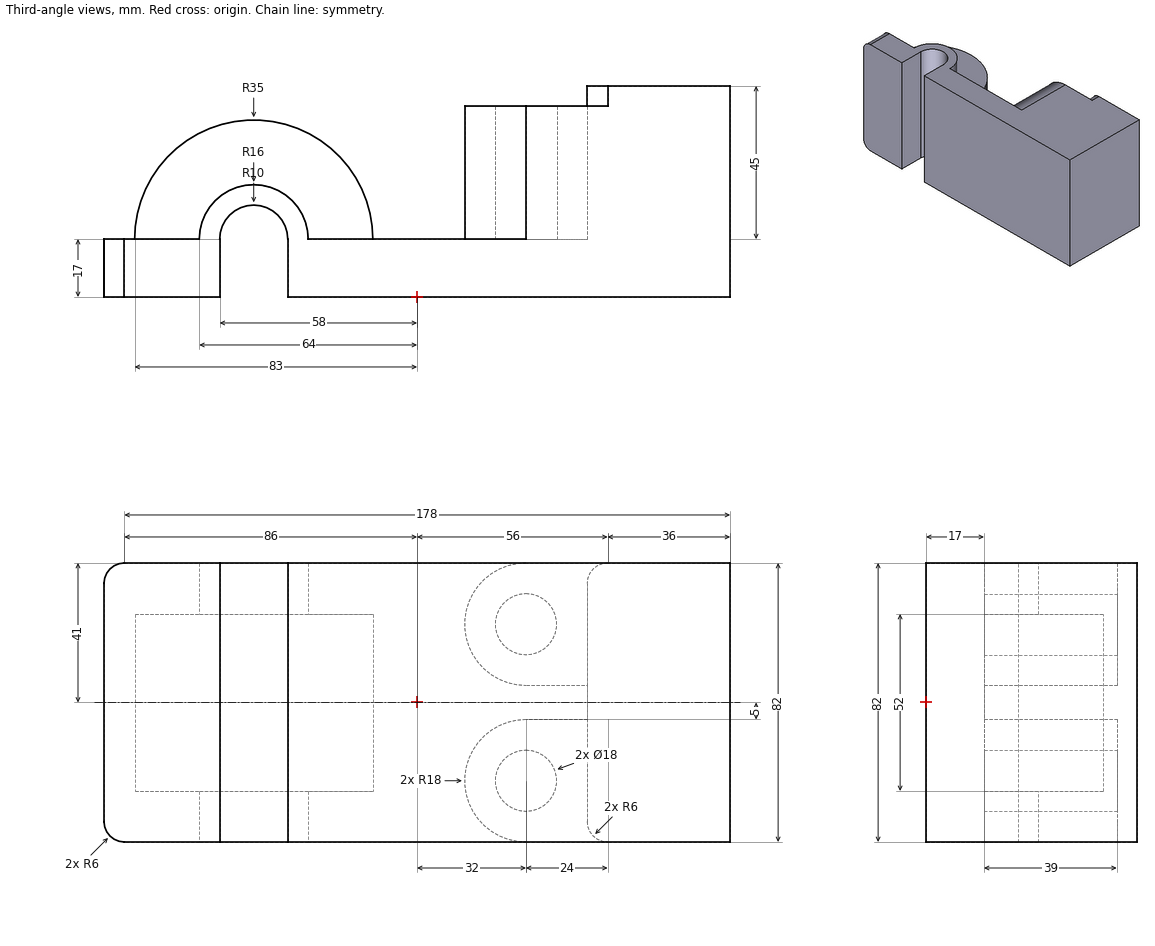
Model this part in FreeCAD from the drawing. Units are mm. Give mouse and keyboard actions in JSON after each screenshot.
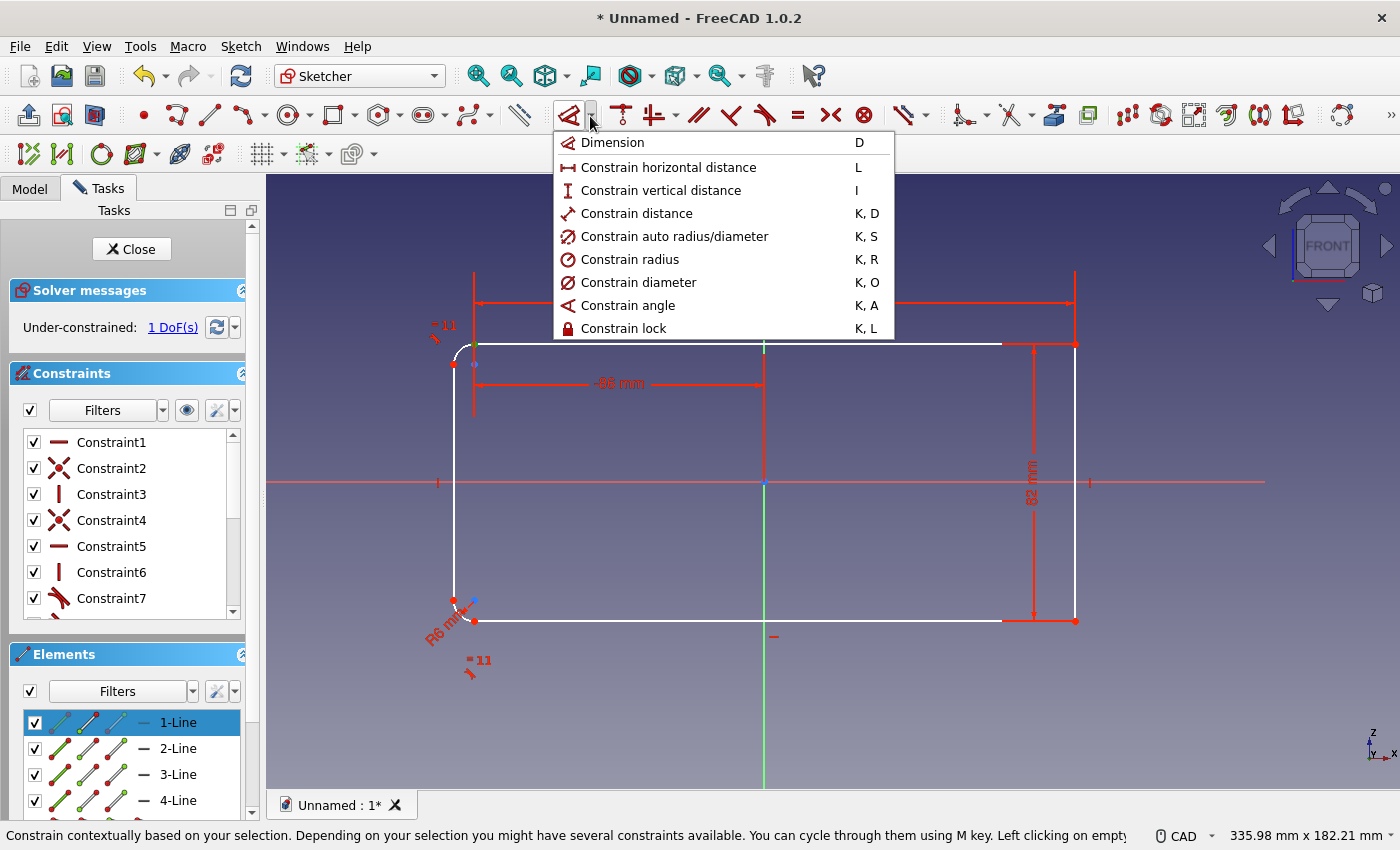
{"action": "left_click", "coordinate": [724, 190]}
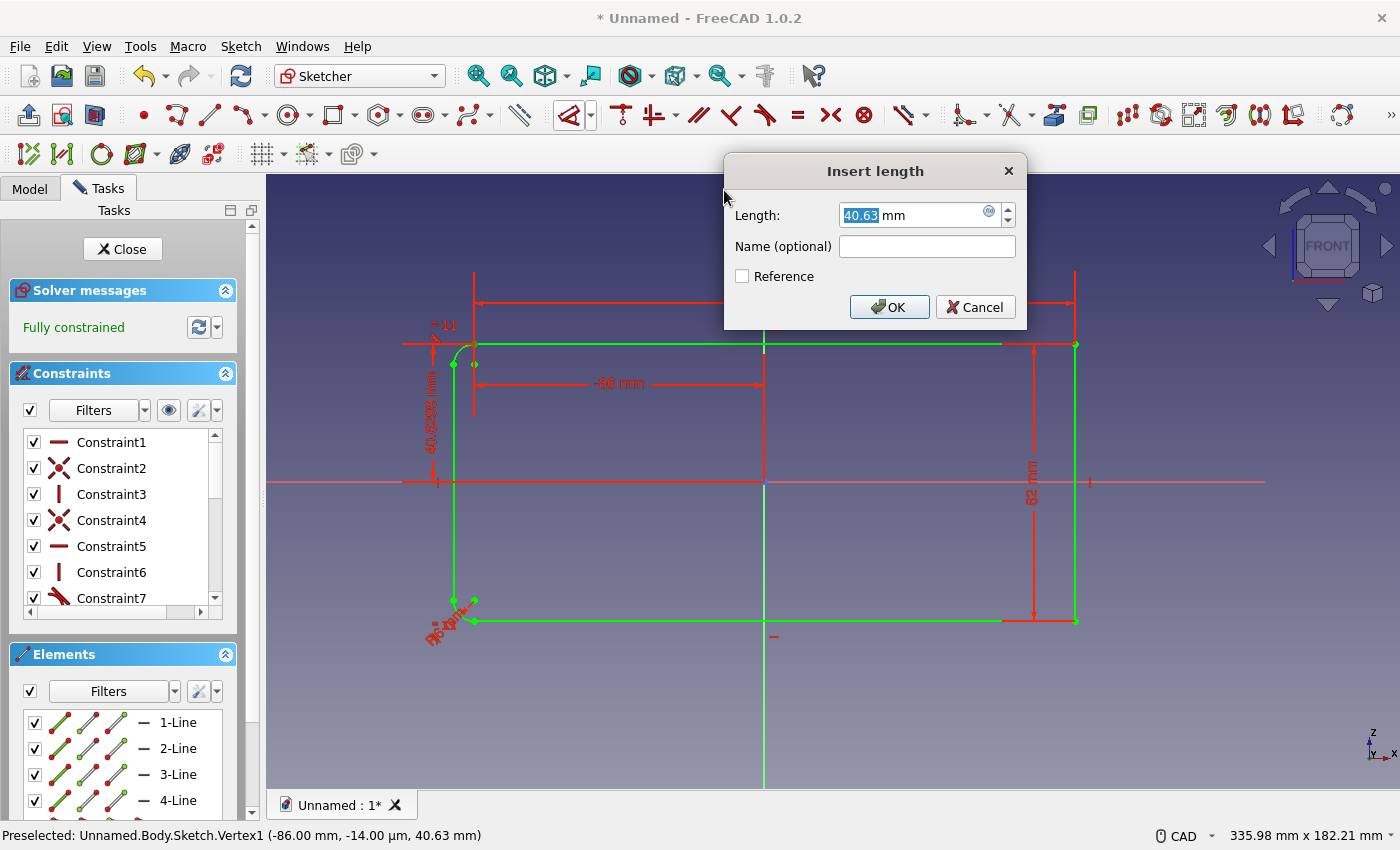
{"action": "type", "text": "41"}
{"action": "key", "text": "Return"}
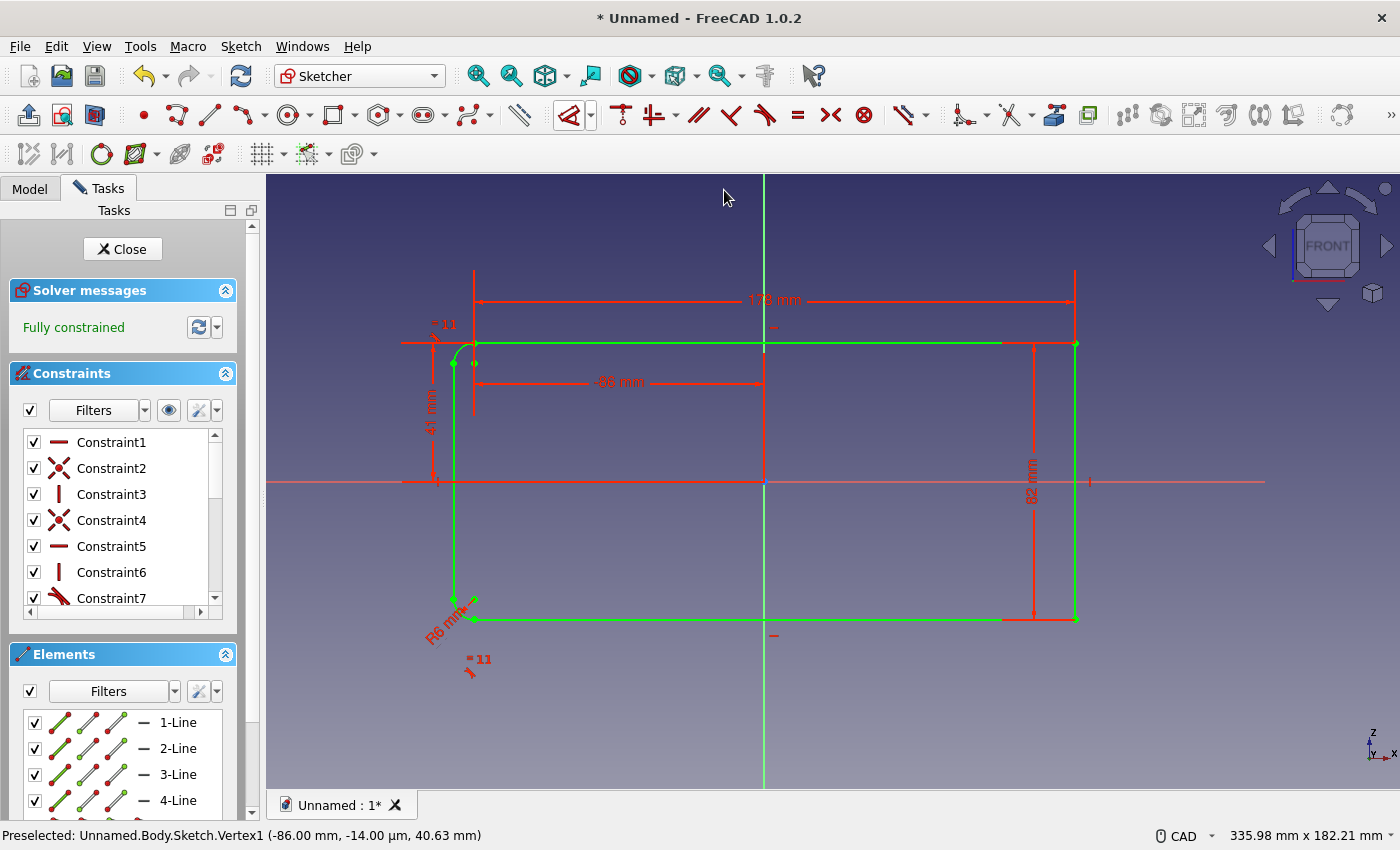
{"action": "left_click", "coordinate": [123, 249]}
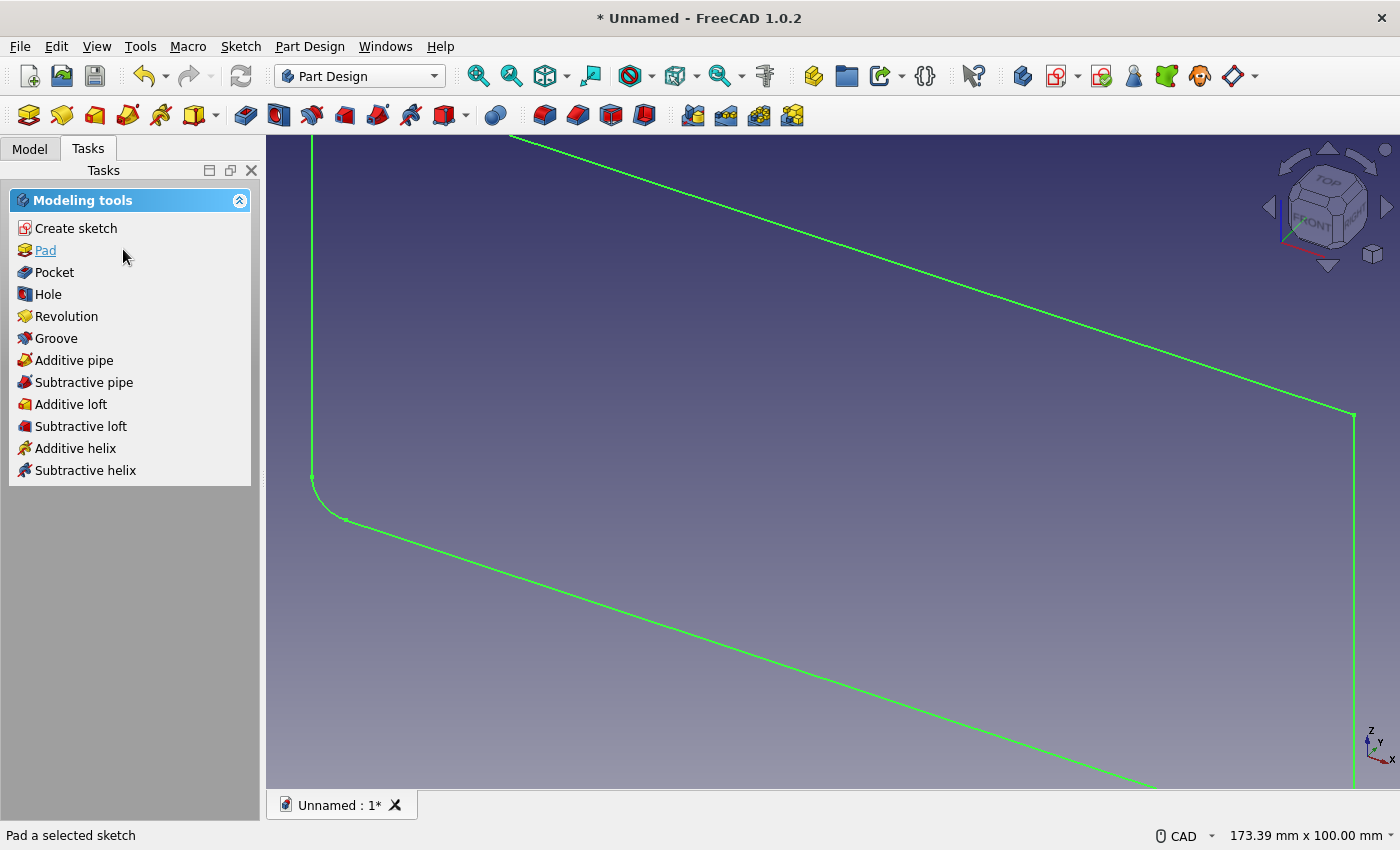
{"action": "left_click", "coordinate": [29, 116]}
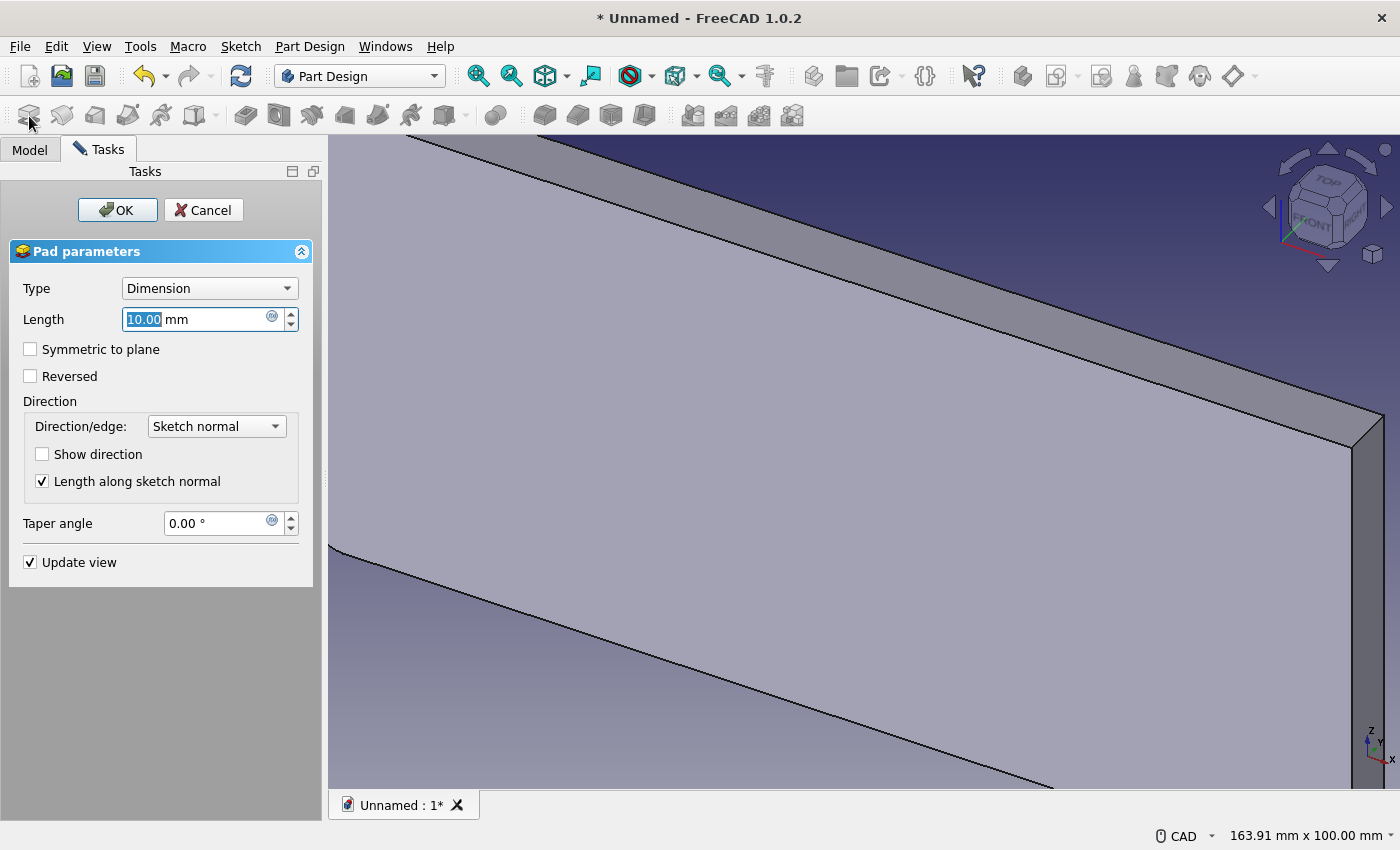
{"action": "type", "text": "17"}
{"action": "key", "text": "Tab"}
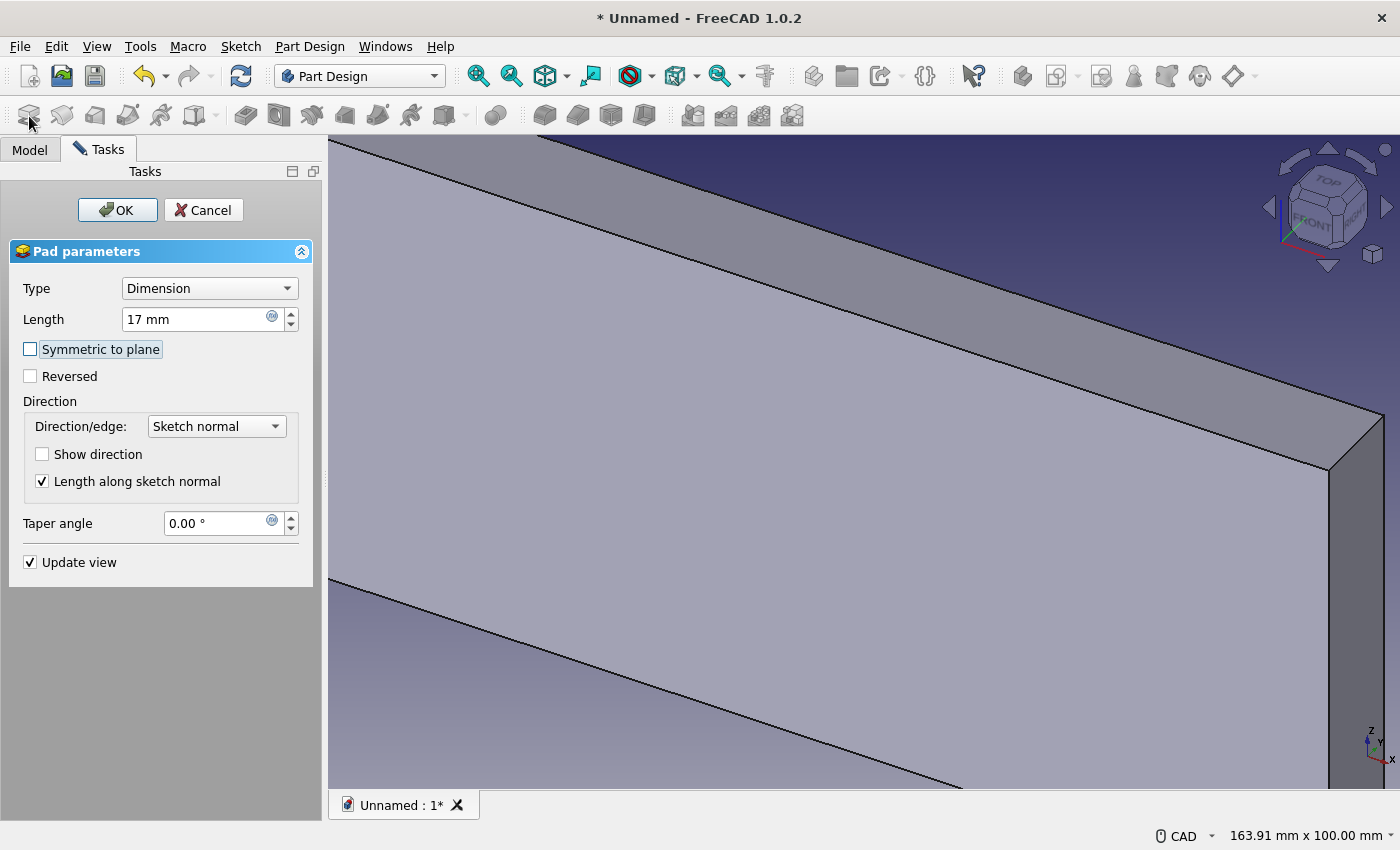
{"action": "left_click", "coordinate": [31, 376]}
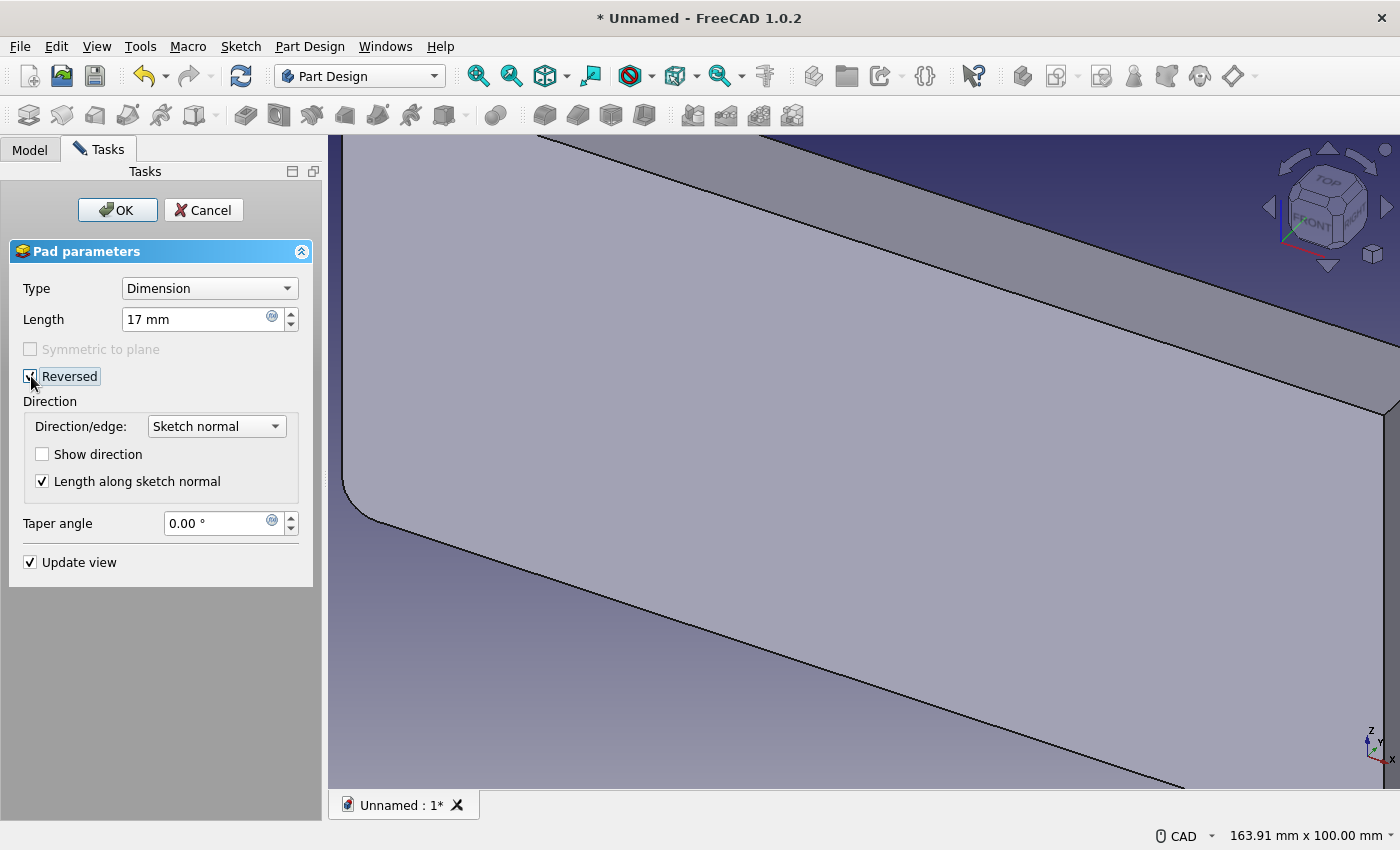
{"action": "left_click", "coordinate": [118, 210]}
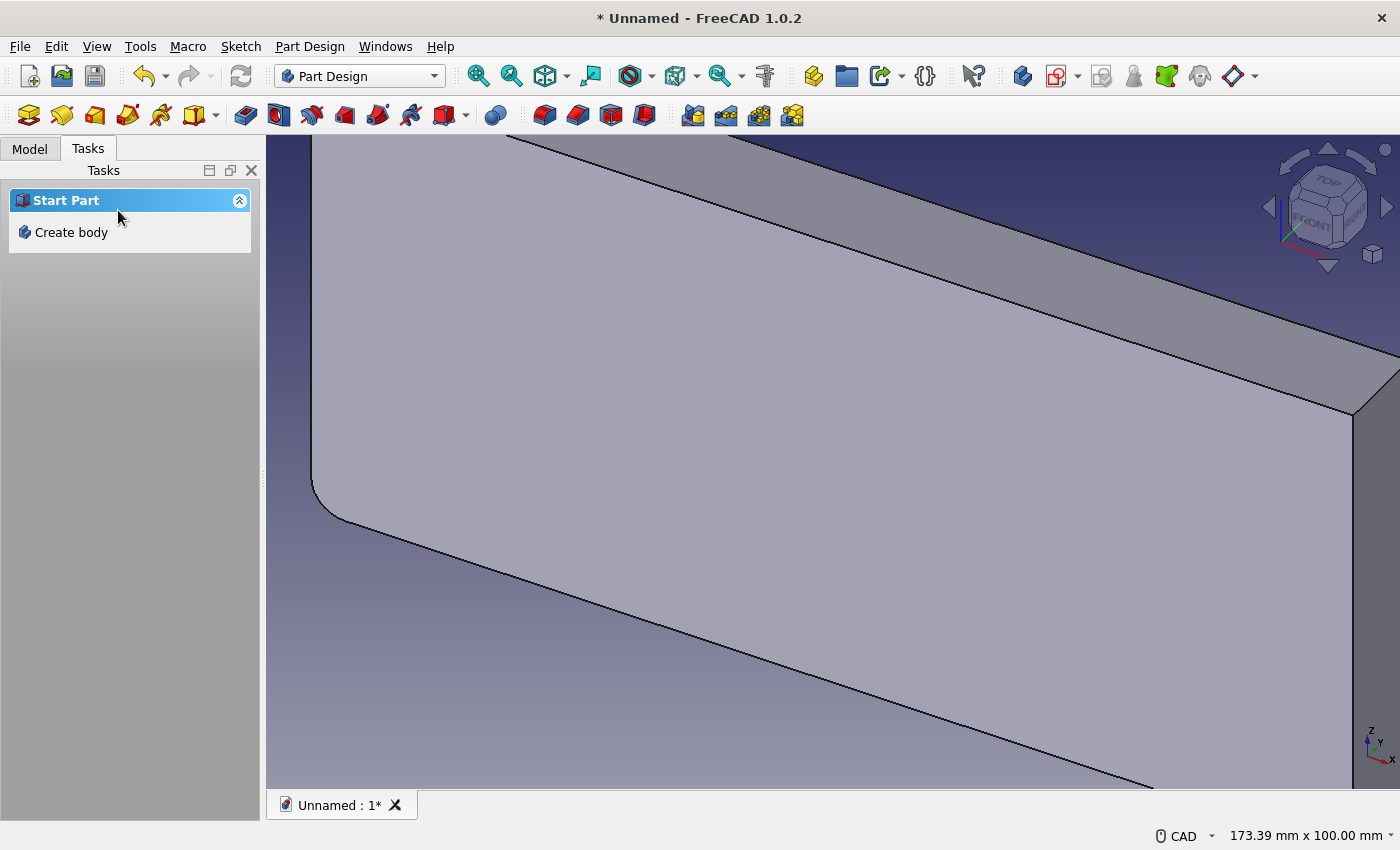
{"action": "left_click", "coordinate": [479, 76]}